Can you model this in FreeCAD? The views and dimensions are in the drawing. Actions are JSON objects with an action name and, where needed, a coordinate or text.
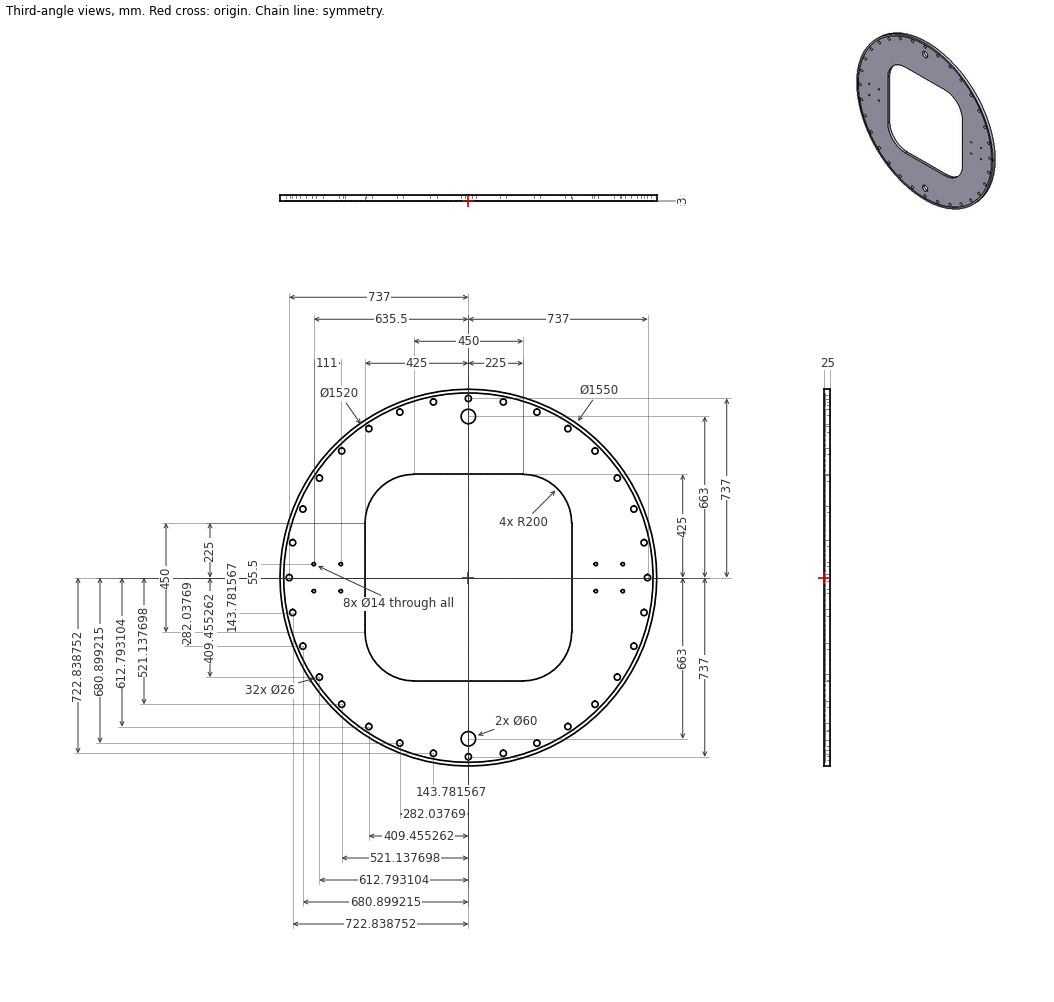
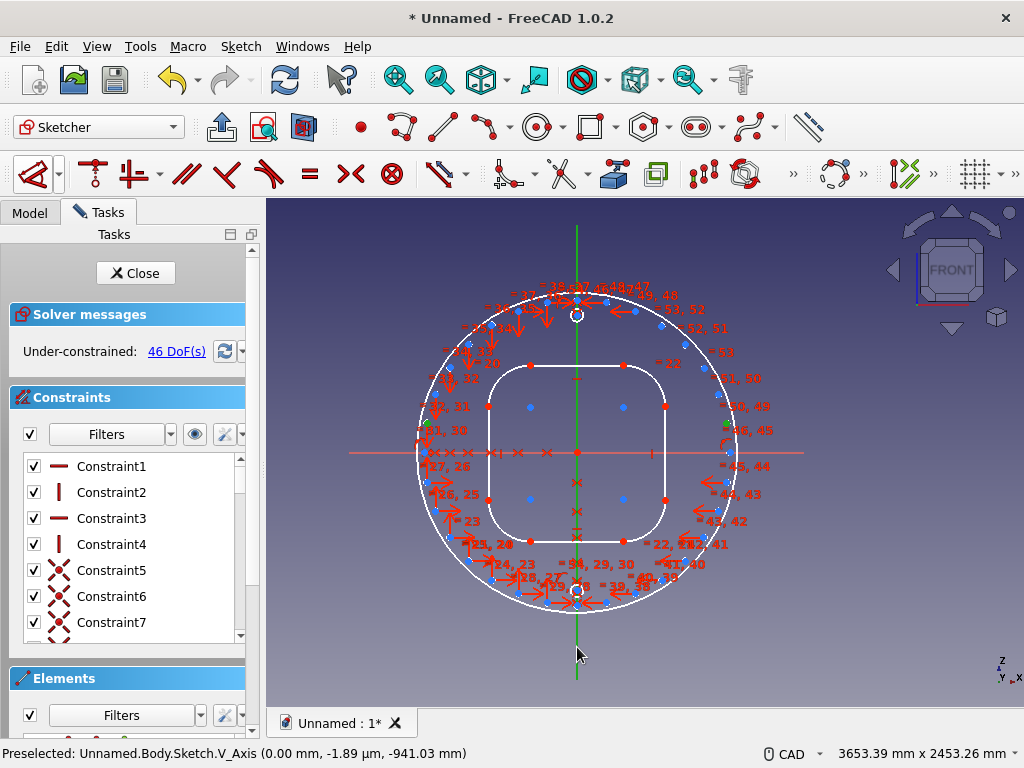
{"action": "left_click", "coordinate": [351, 174]}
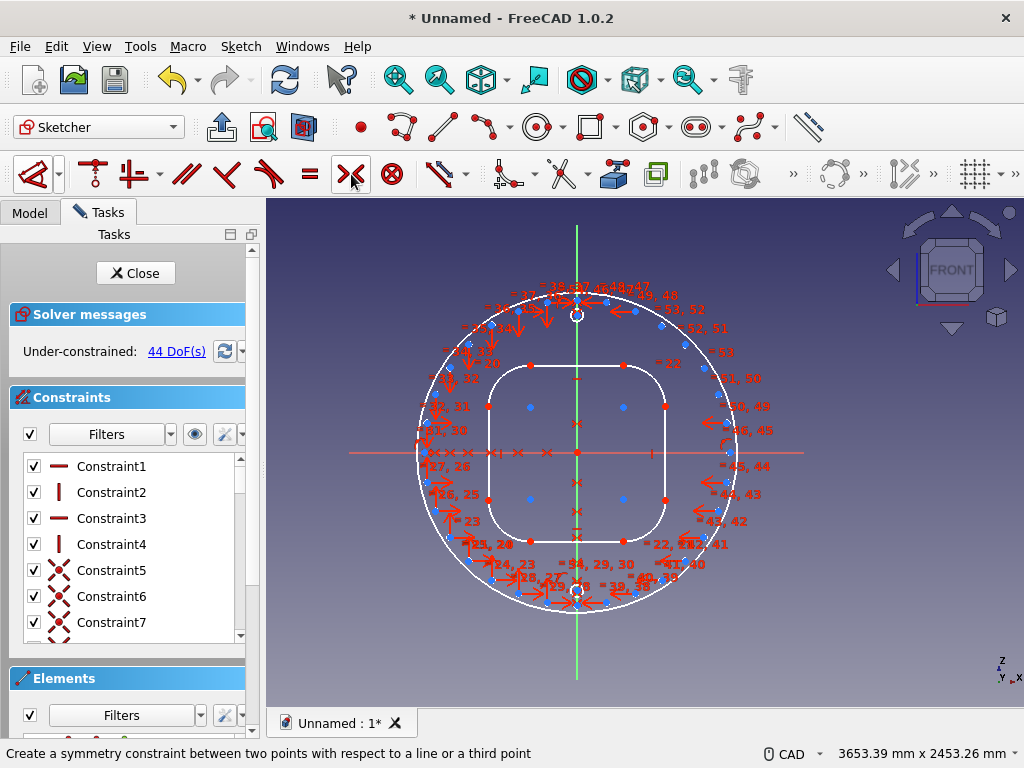
{"action": "left_click", "coordinate": [436, 394]}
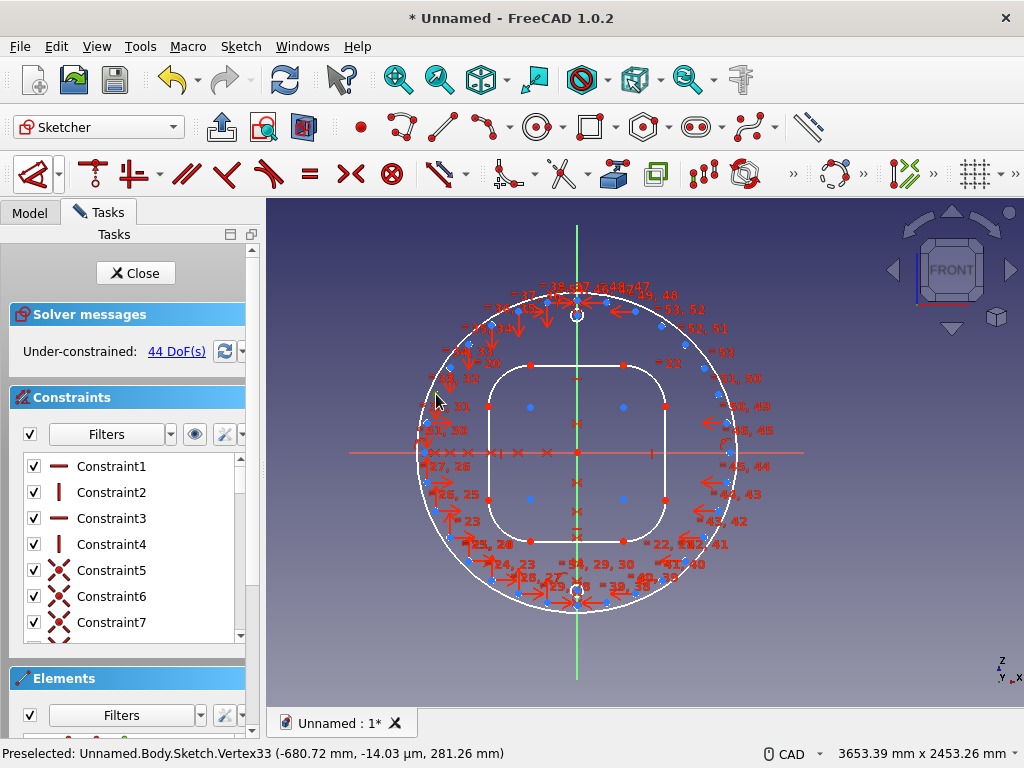
{"action": "left_click", "coordinate": [718, 395]}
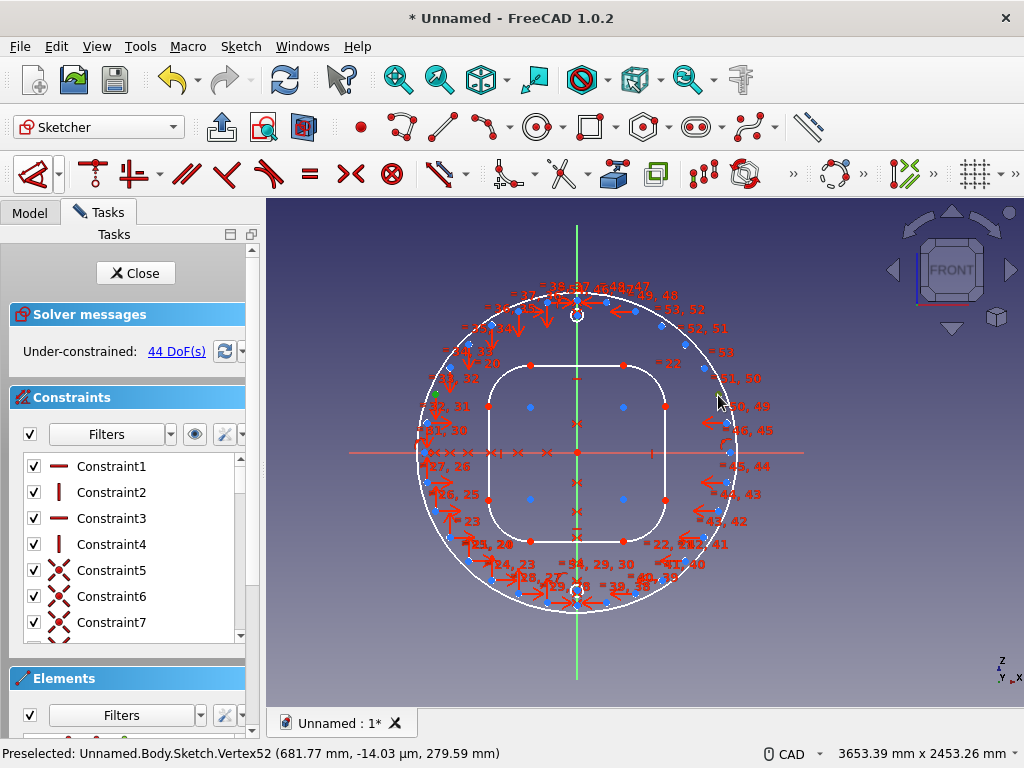
{"action": "left_click", "coordinate": [577, 647]}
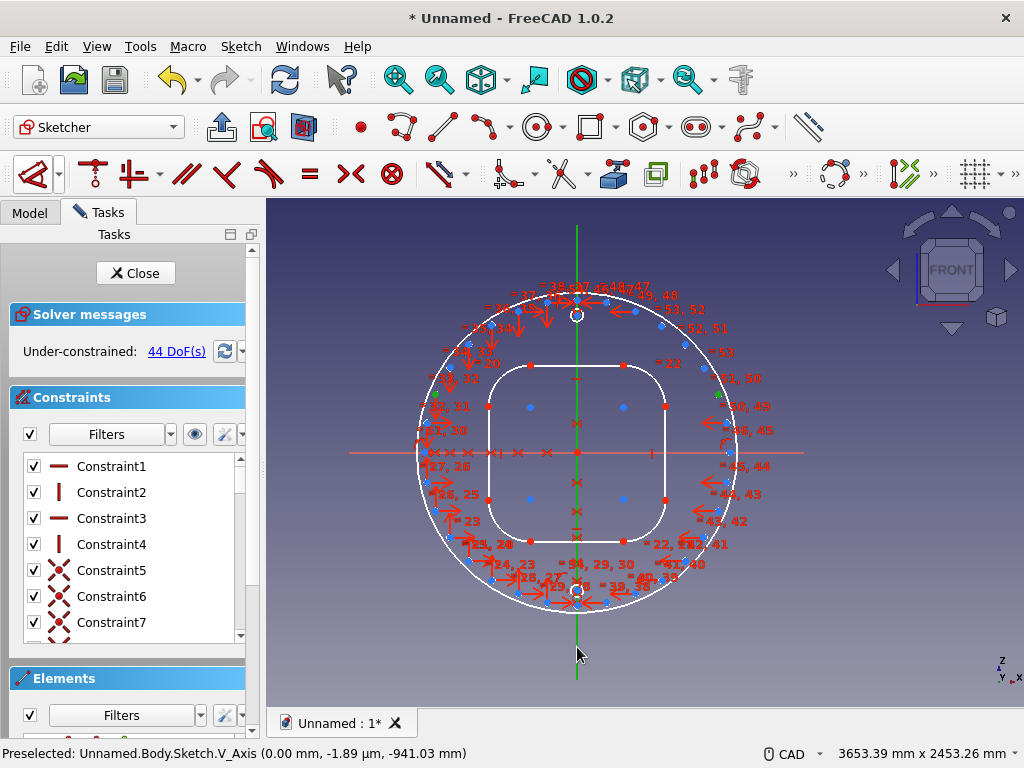
{"action": "left_click", "coordinate": [351, 174]}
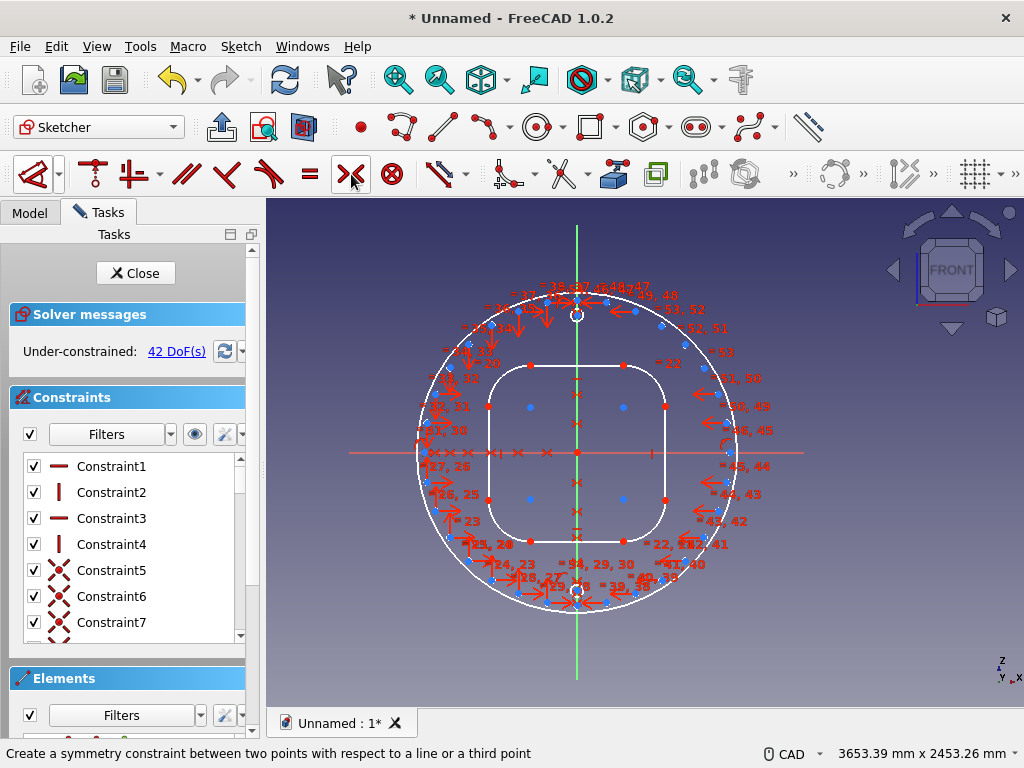
{"action": "left_click", "coordinate": [469, 344]}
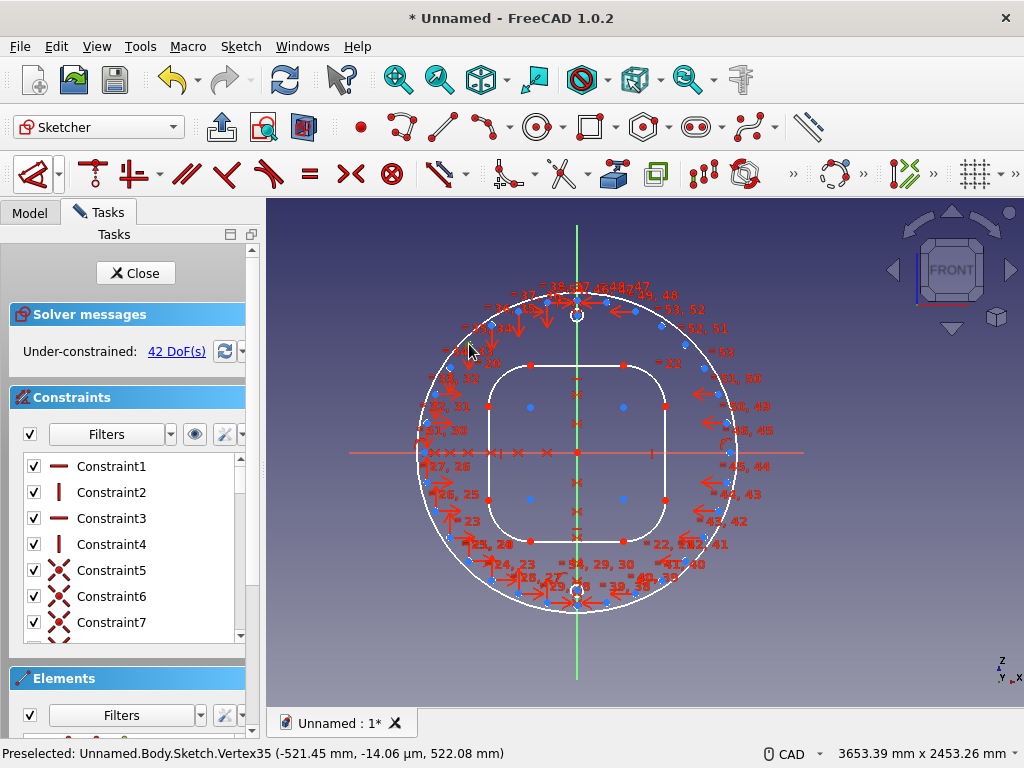
{"action": "left_click", "coordinate": [685, 345]}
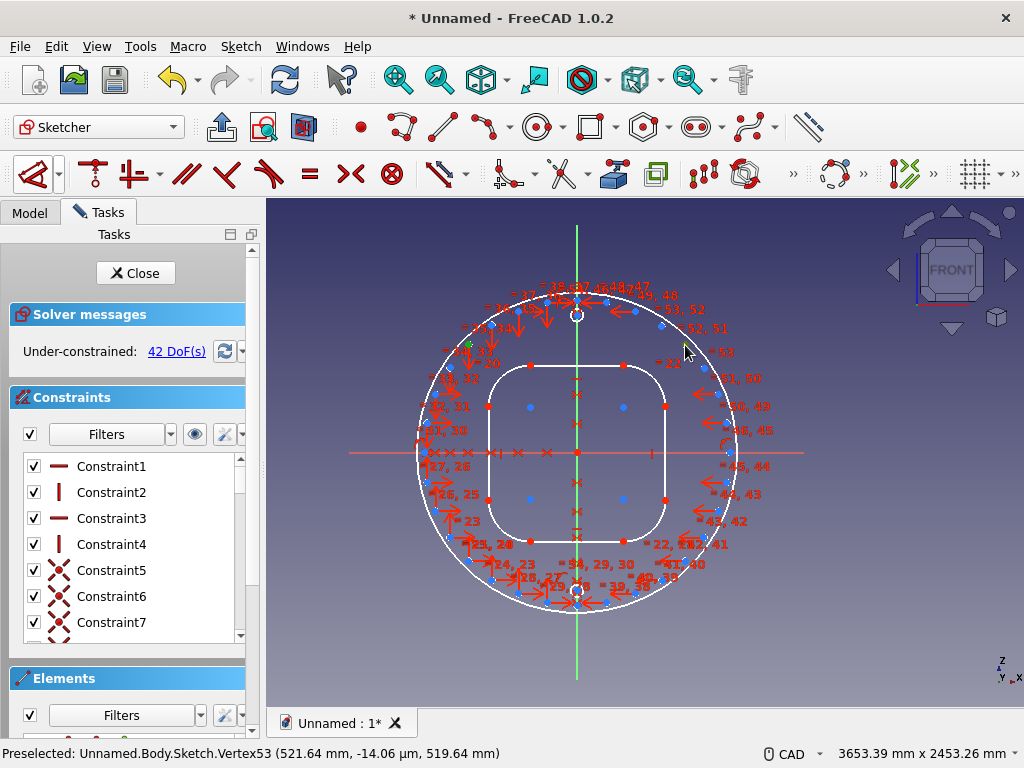
{"action": "left_click", "coordinate": [577, 647]}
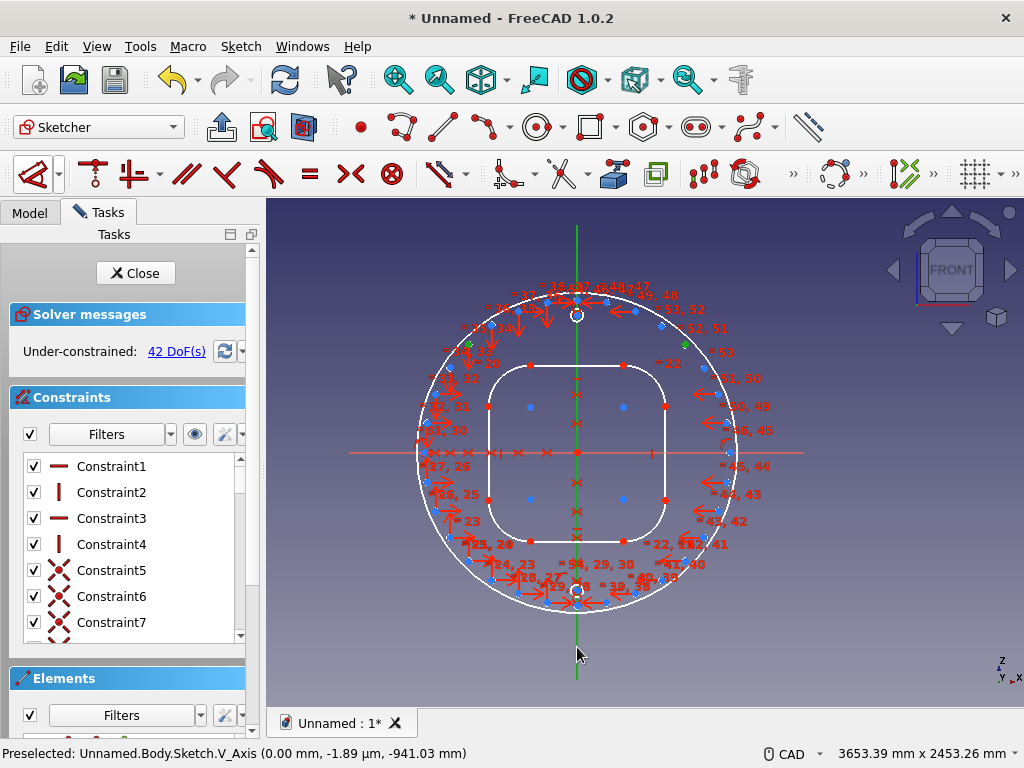
{"action": "left_click", "coordinate": [351, 174]}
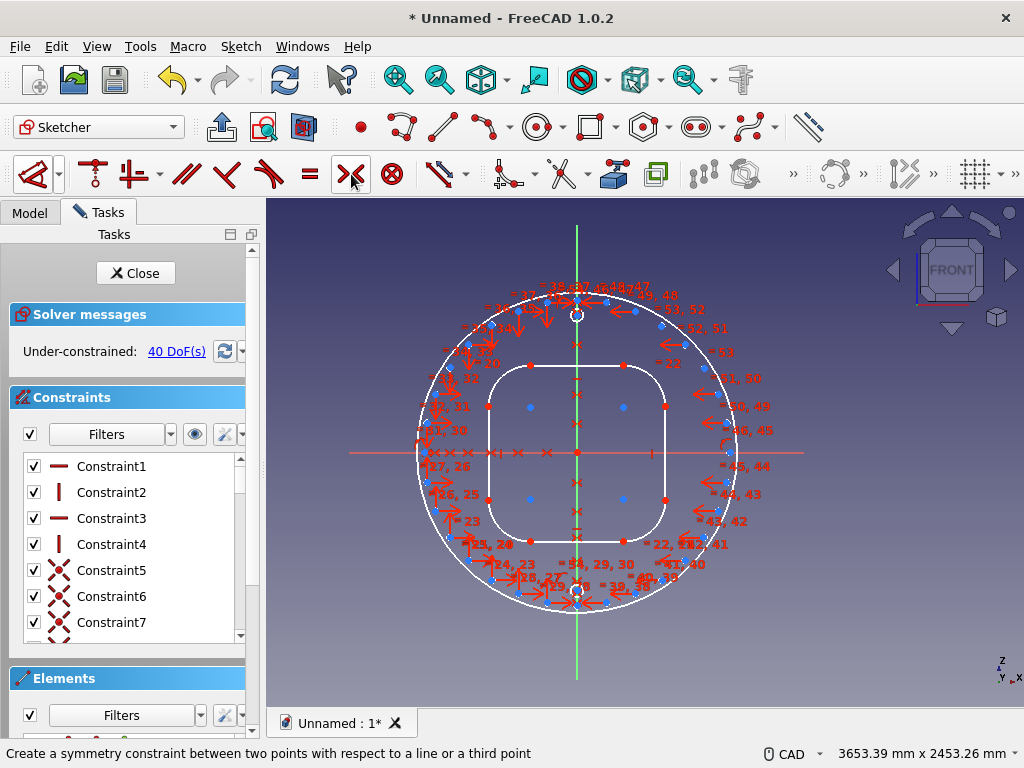
{"action": "left_click", "coordinate": [492, 325]}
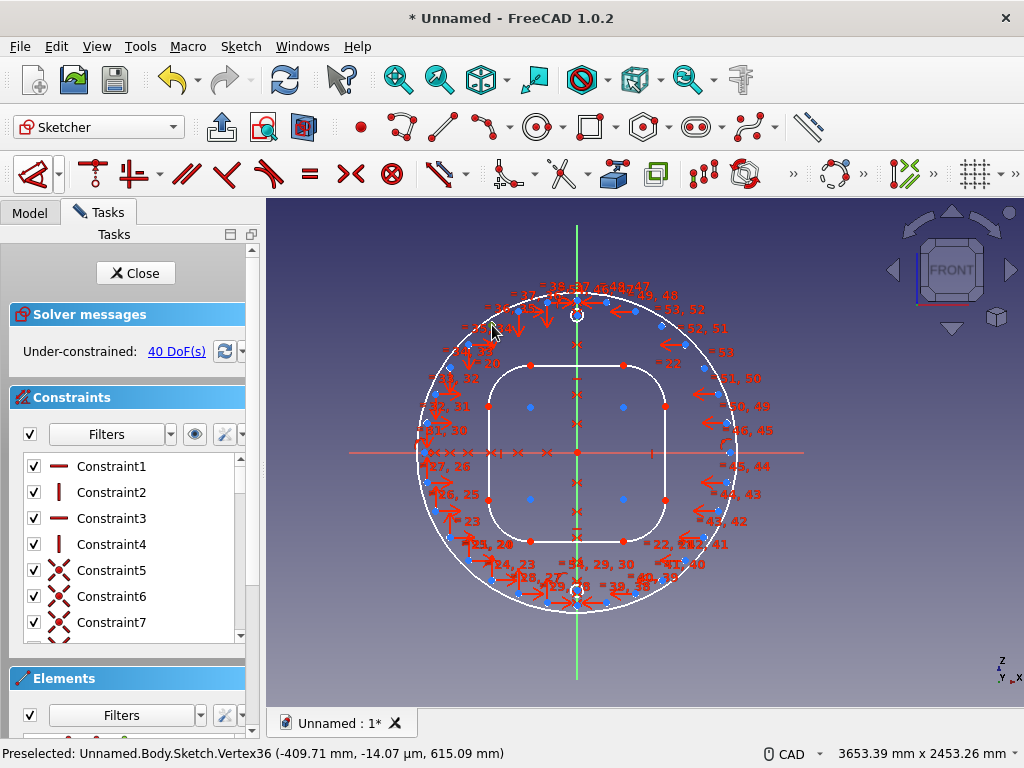
{"action": "left_click", "coordinate": [662, 326]}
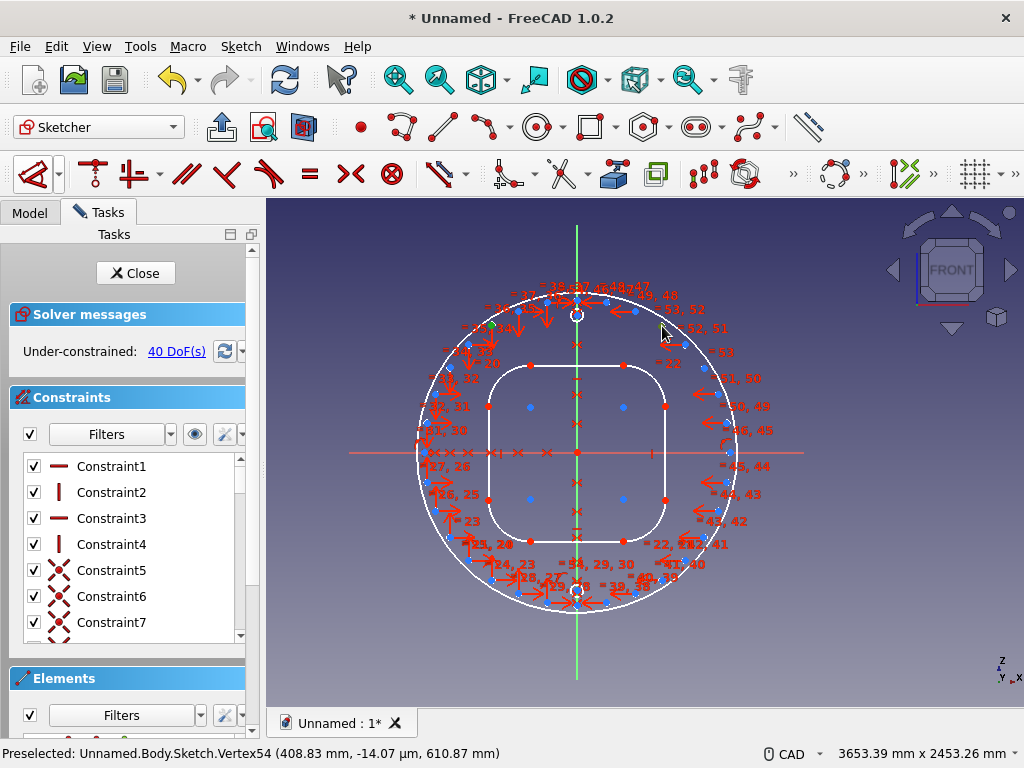
{"action": "left_click", "coordinate": [577, 647]}